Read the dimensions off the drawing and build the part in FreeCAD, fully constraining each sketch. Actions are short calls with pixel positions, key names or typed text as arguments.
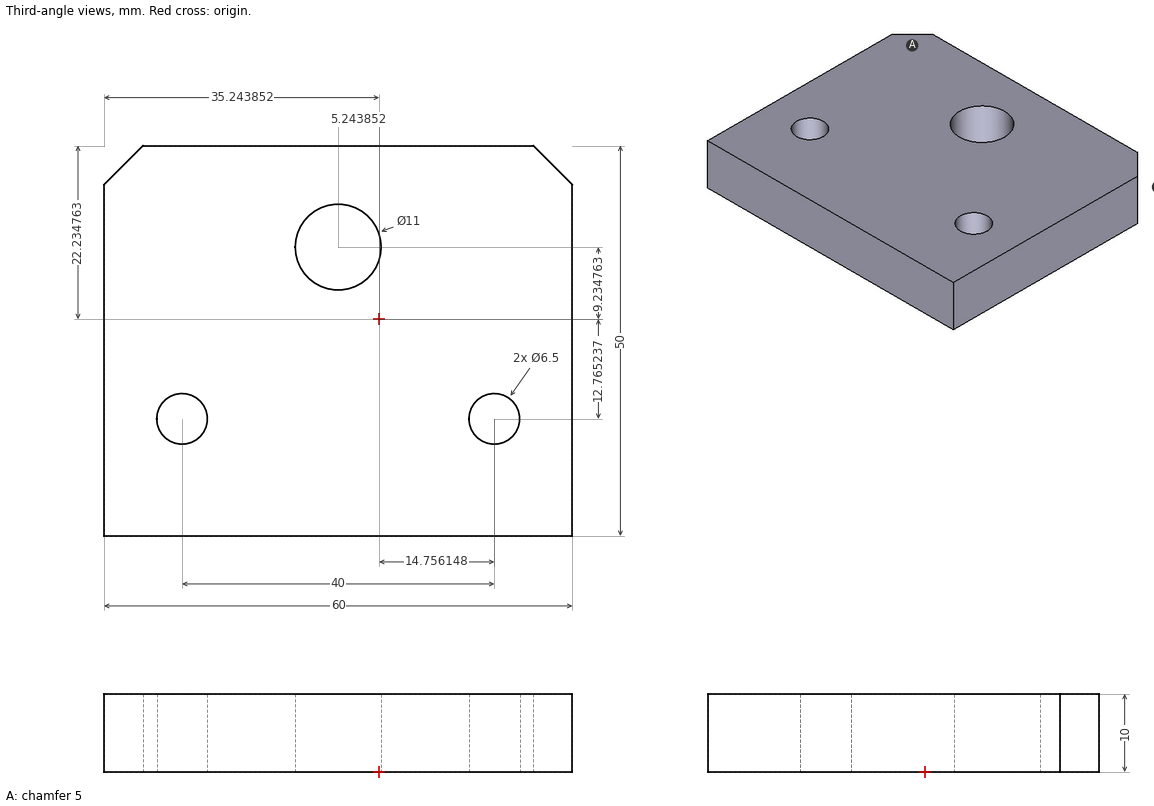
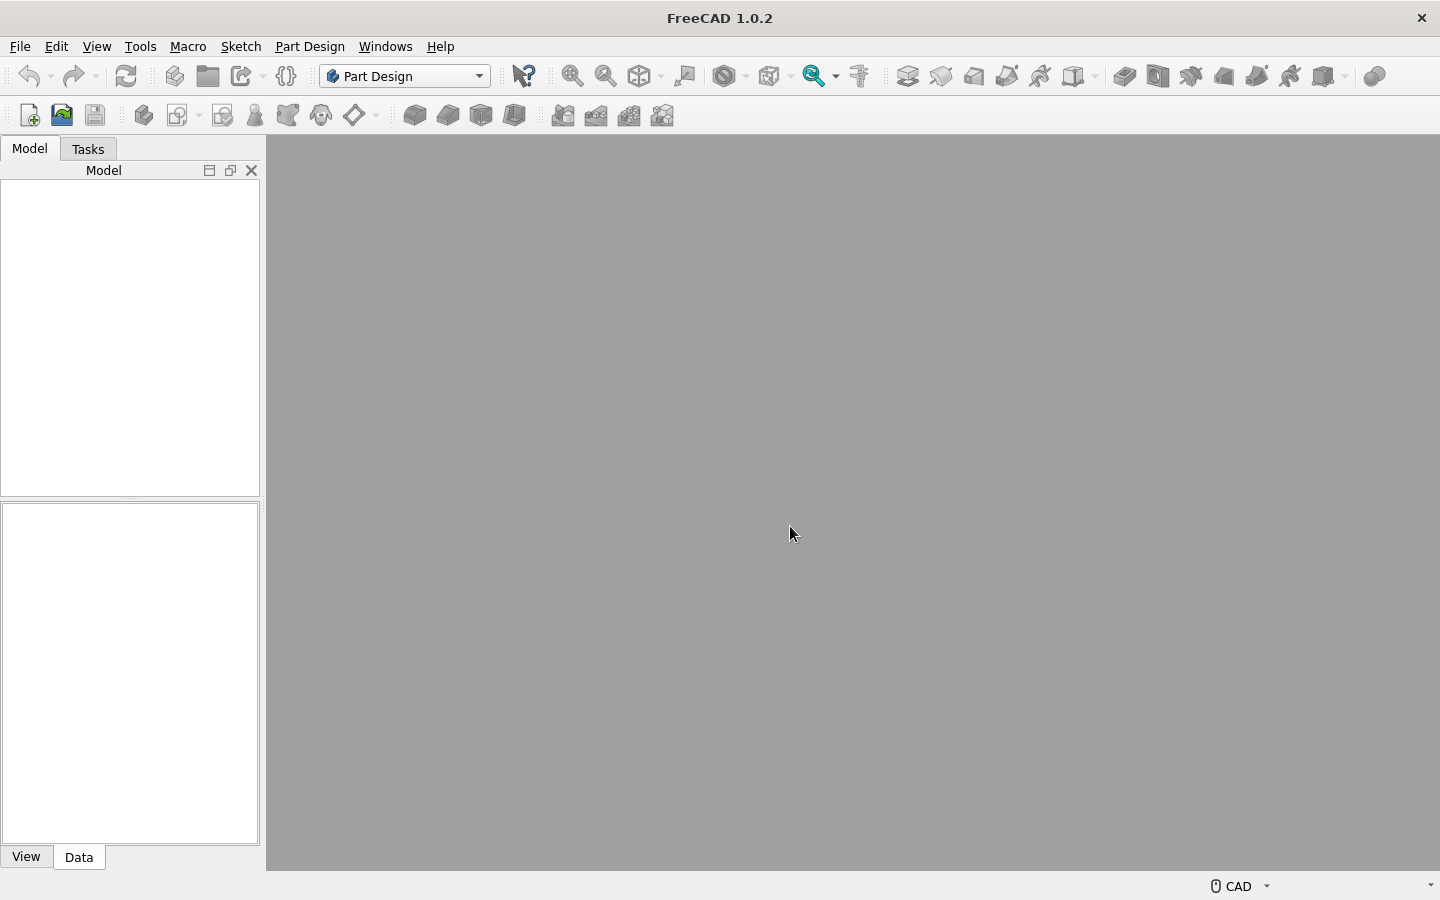
key(ctrl+n)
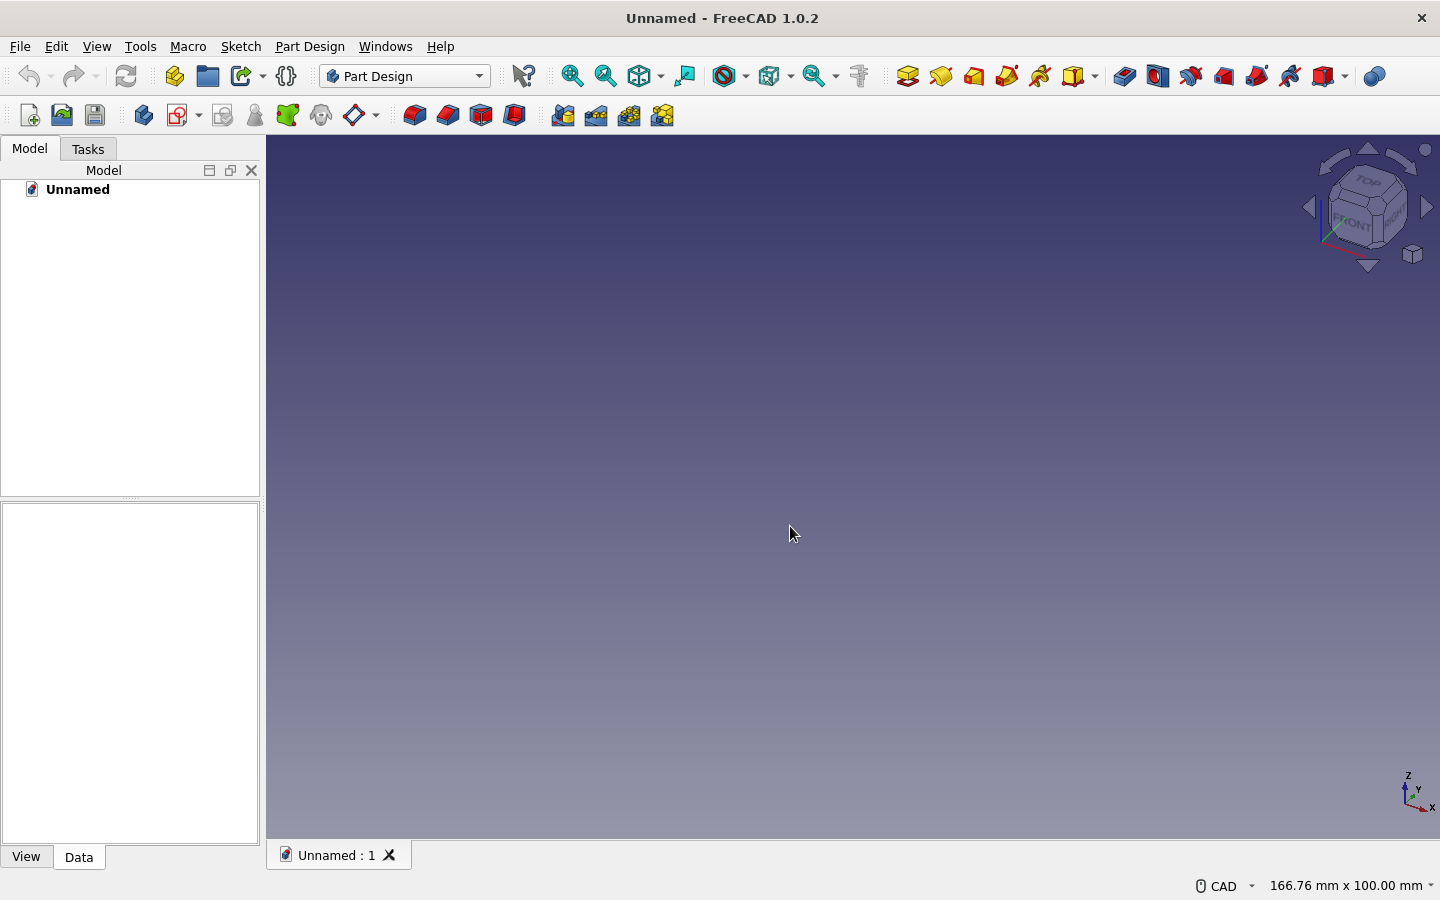
click(176, 116)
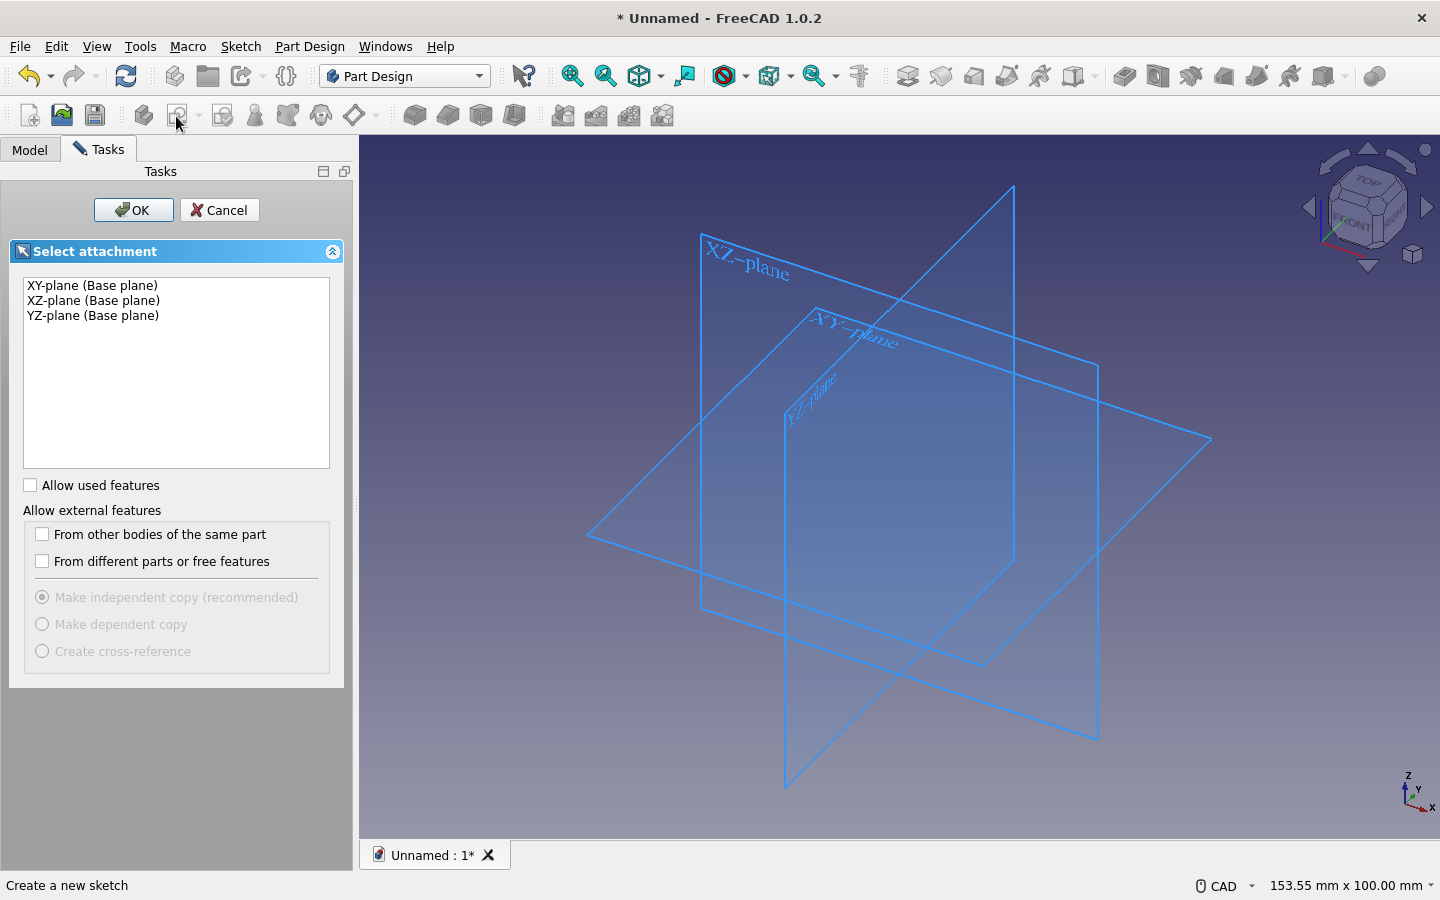
click(84, 286)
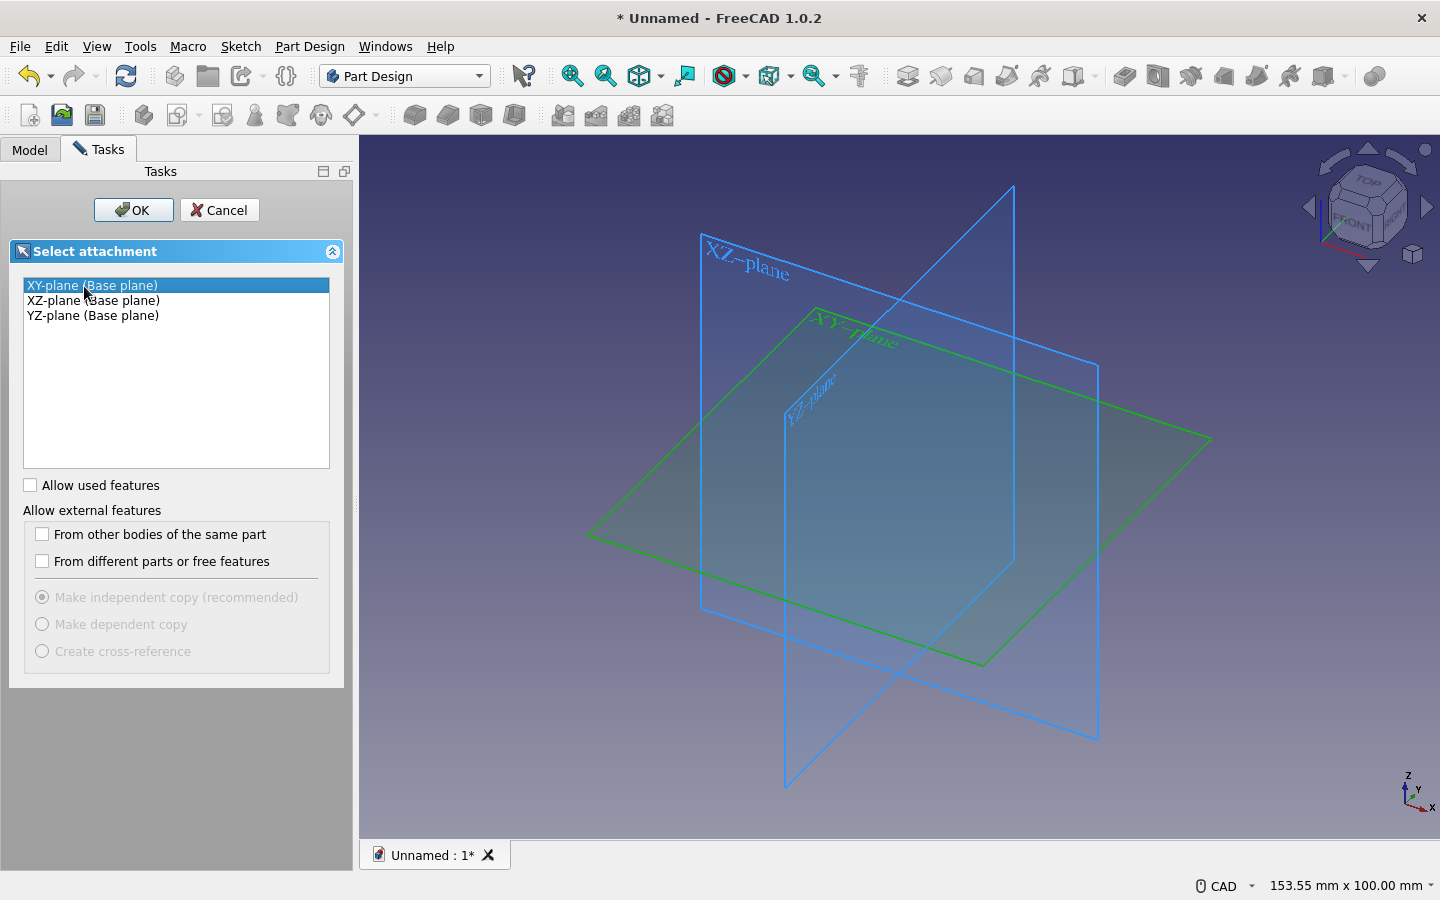
click(134, 210)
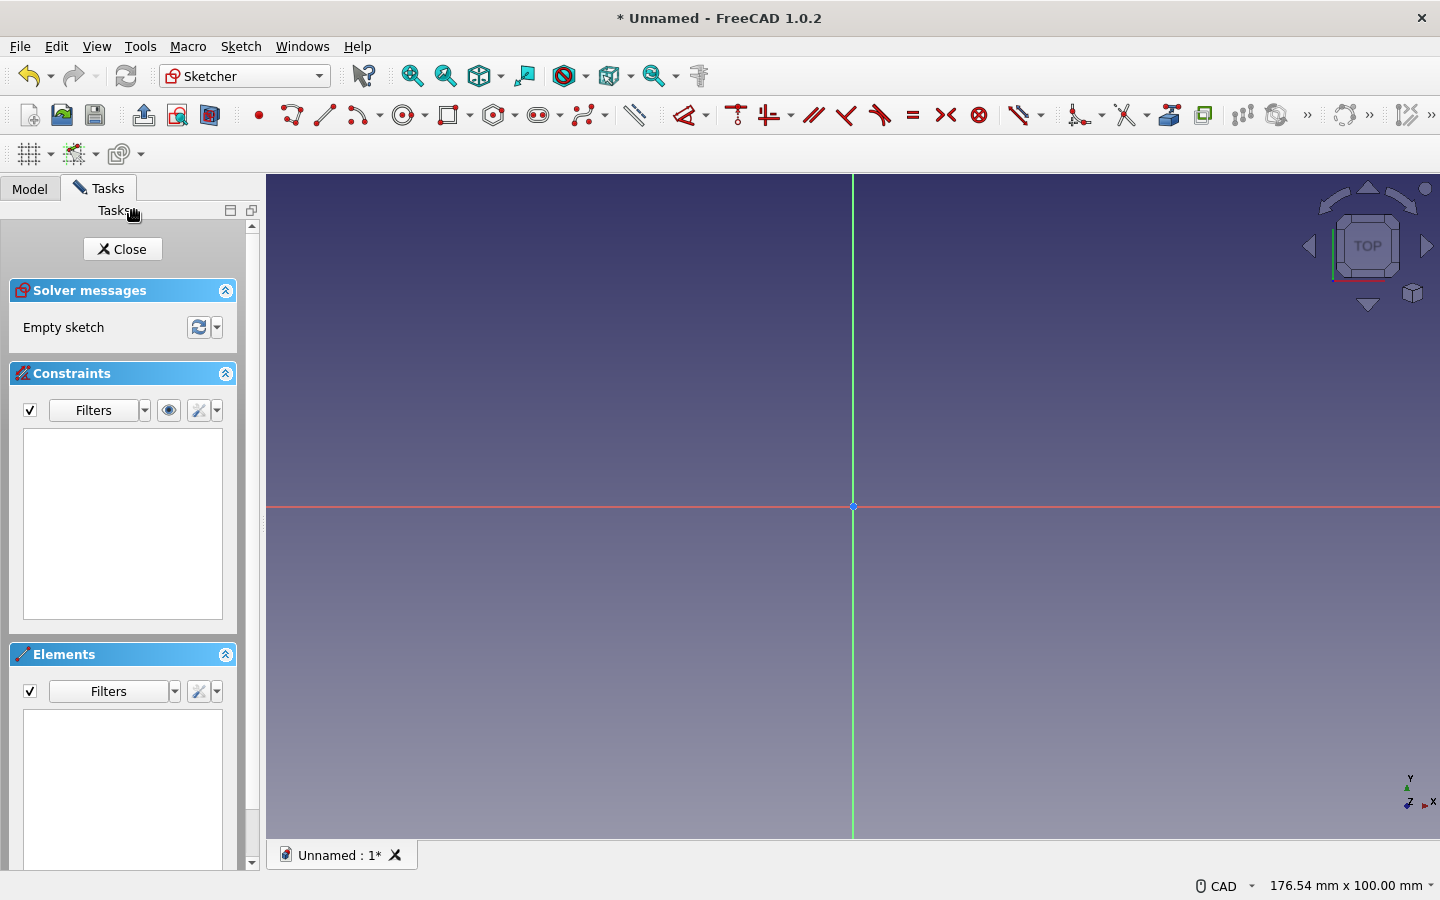
key(g)
key(r)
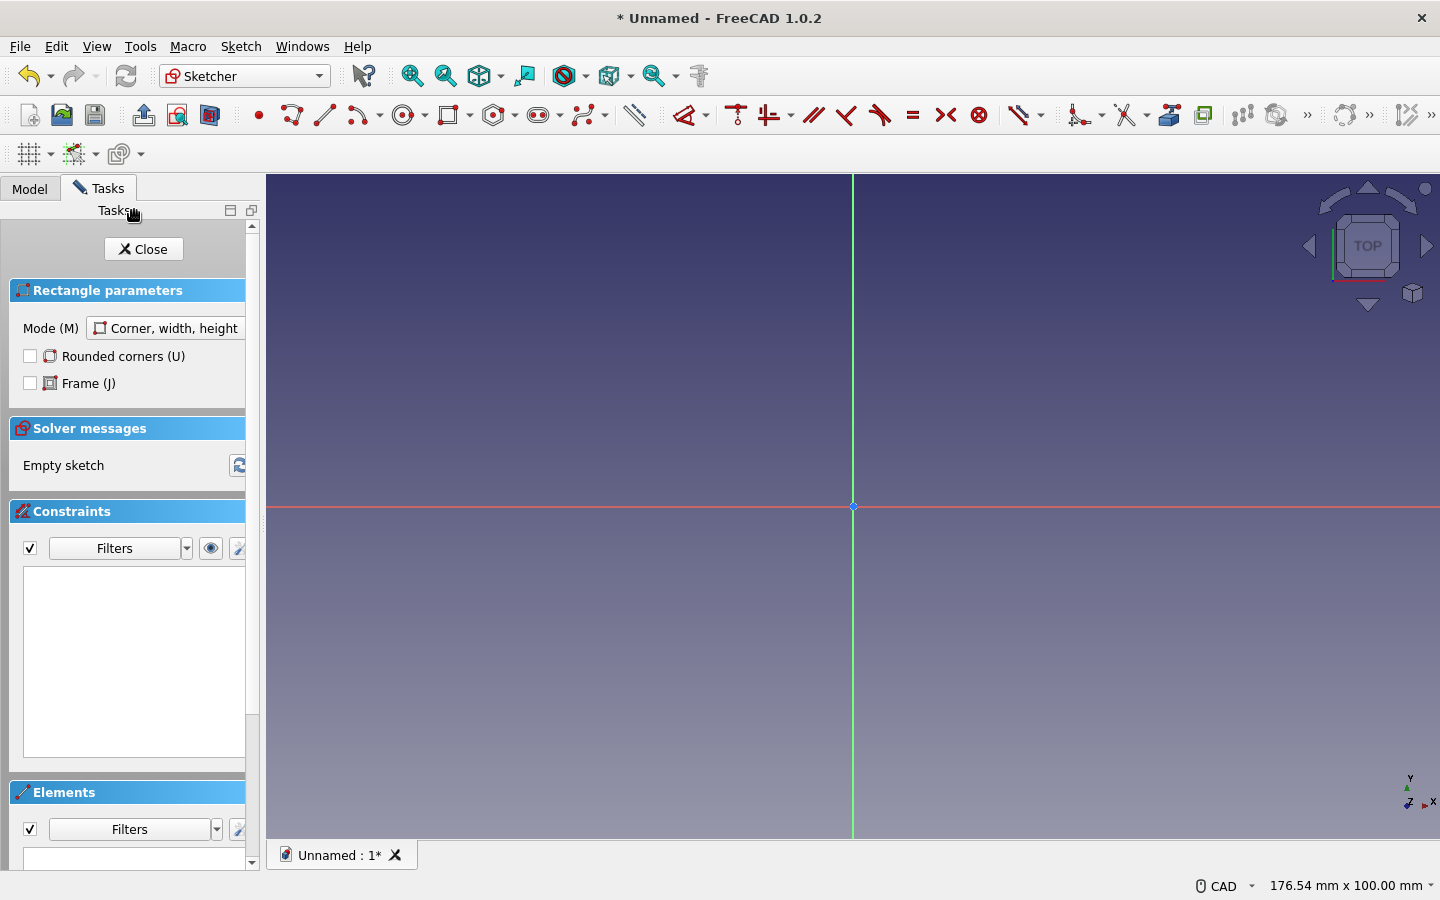
click(619, 359)
move(1018, 691)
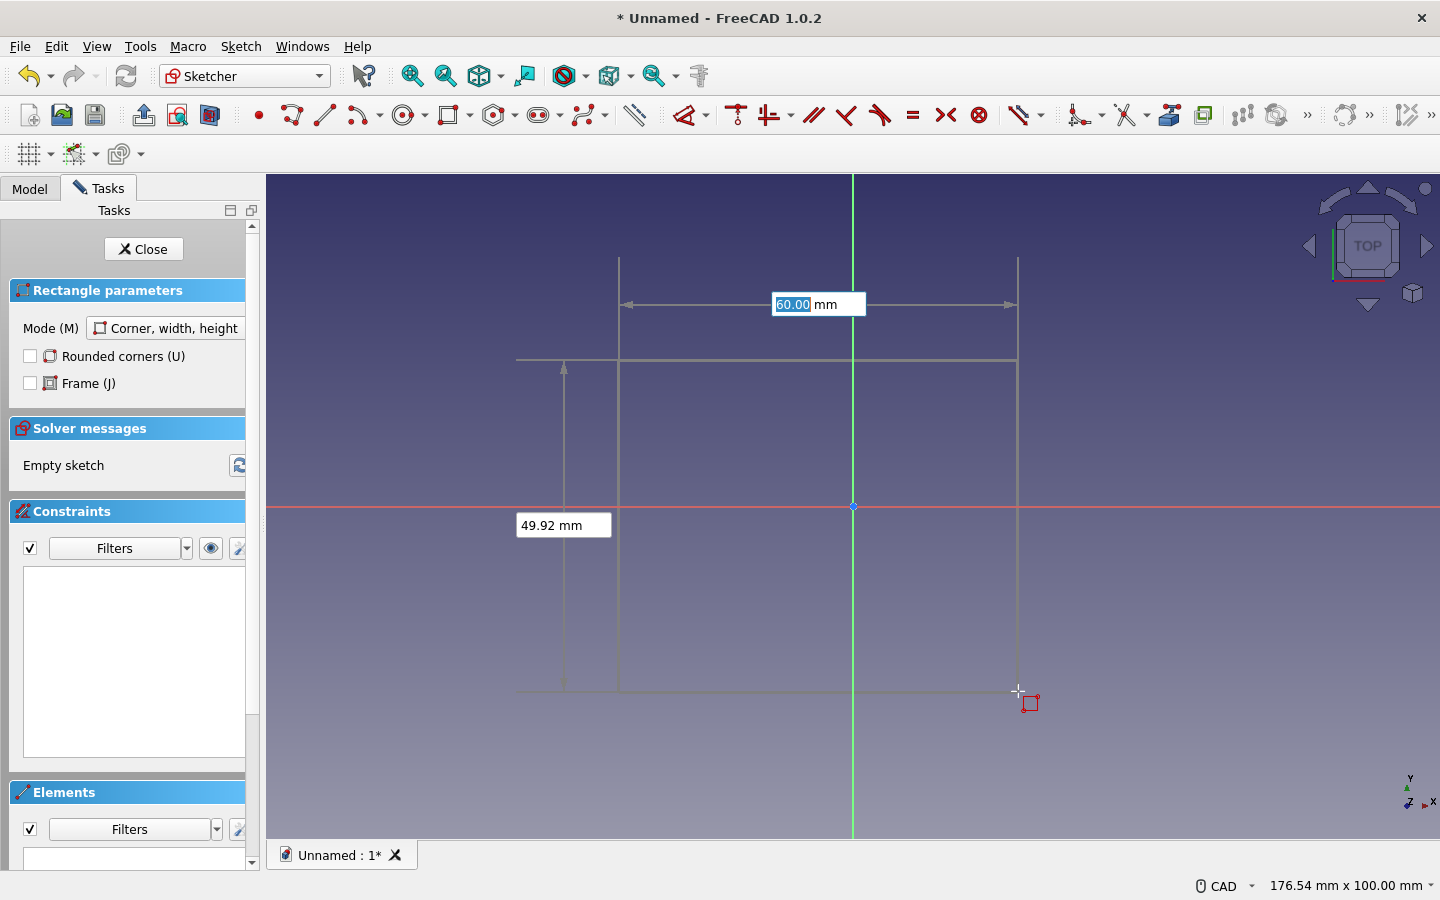
text(60)
key(Tab)
text(50)
key(Return)
key(Escape)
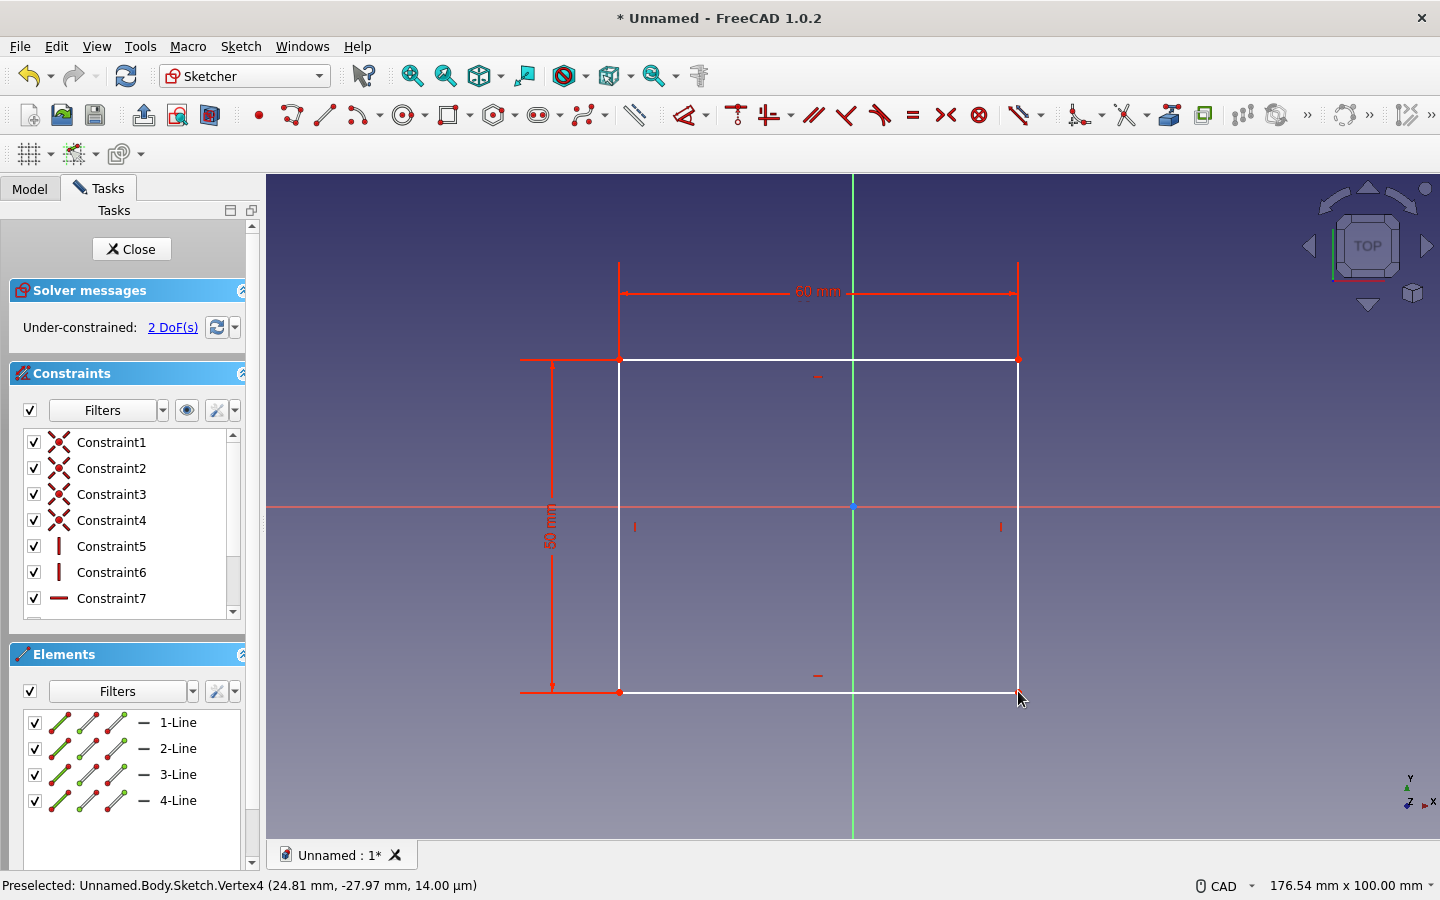
key(d)